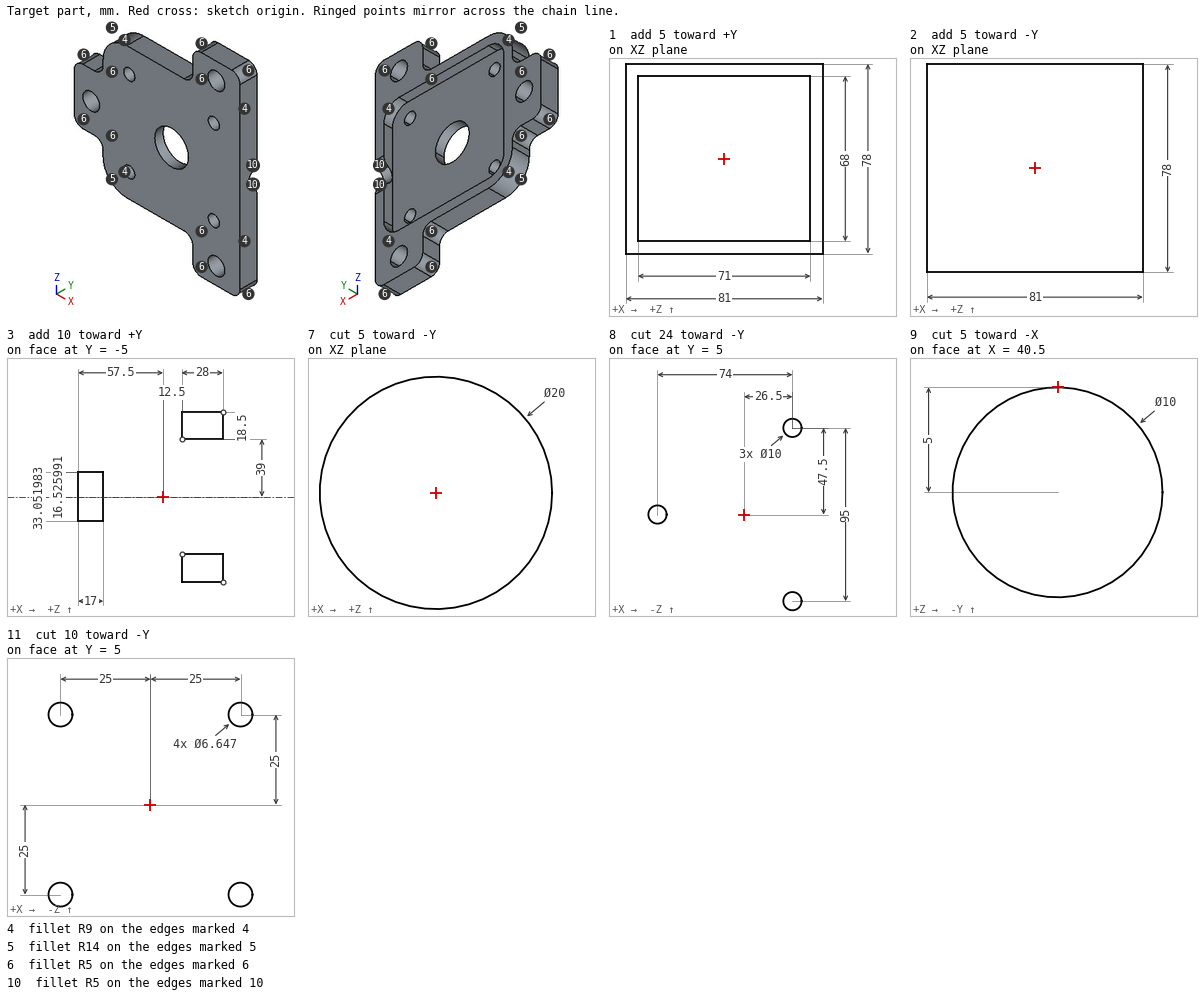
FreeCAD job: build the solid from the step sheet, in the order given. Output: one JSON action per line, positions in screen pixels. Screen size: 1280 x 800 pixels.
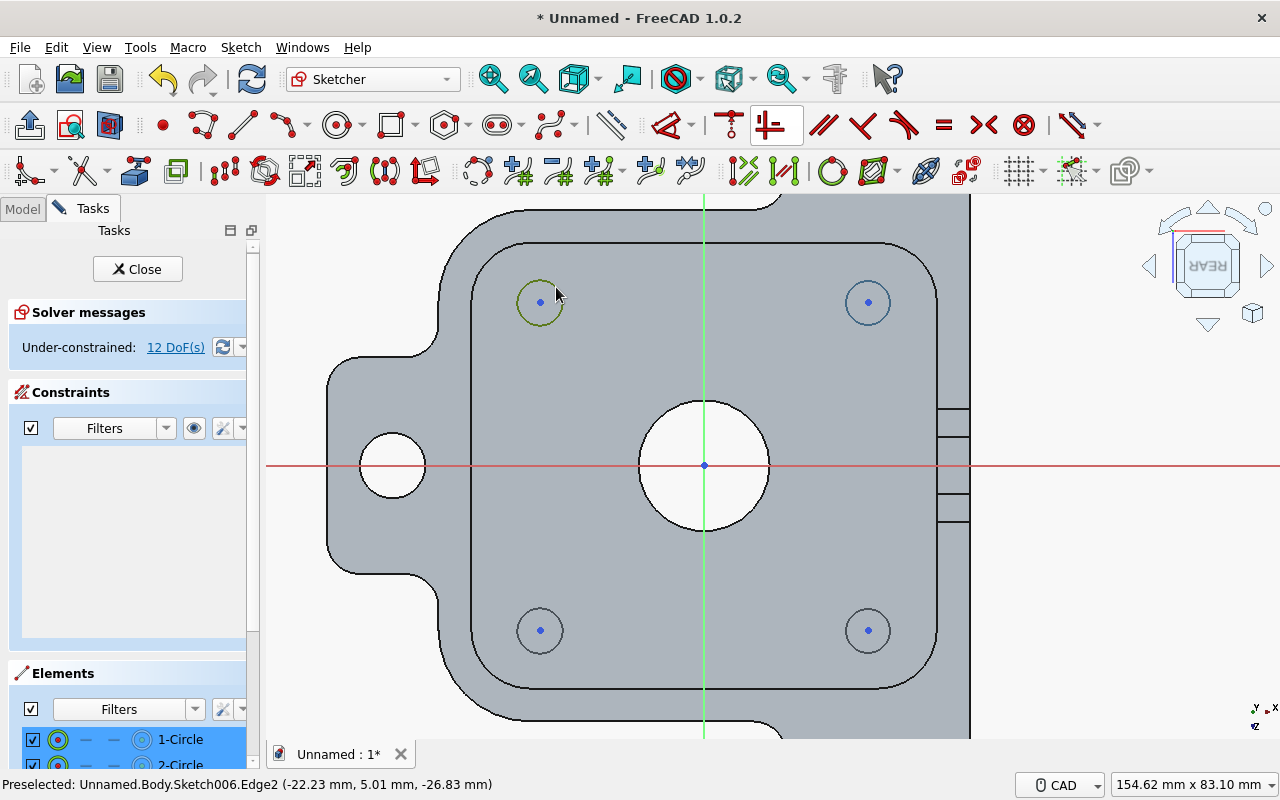
{"action": "left_click", "coordinate": [556, 615]}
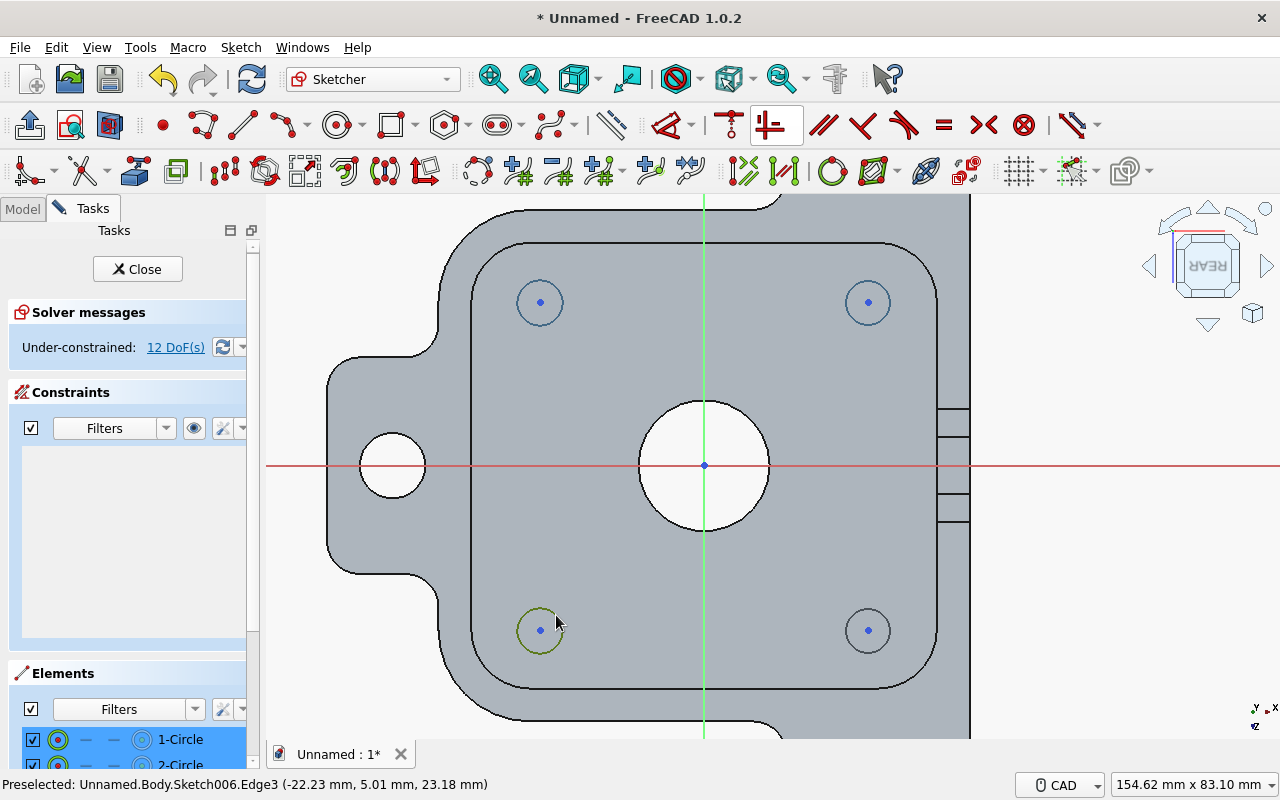
{"action": "left_click", "coordinate": [883, 615]}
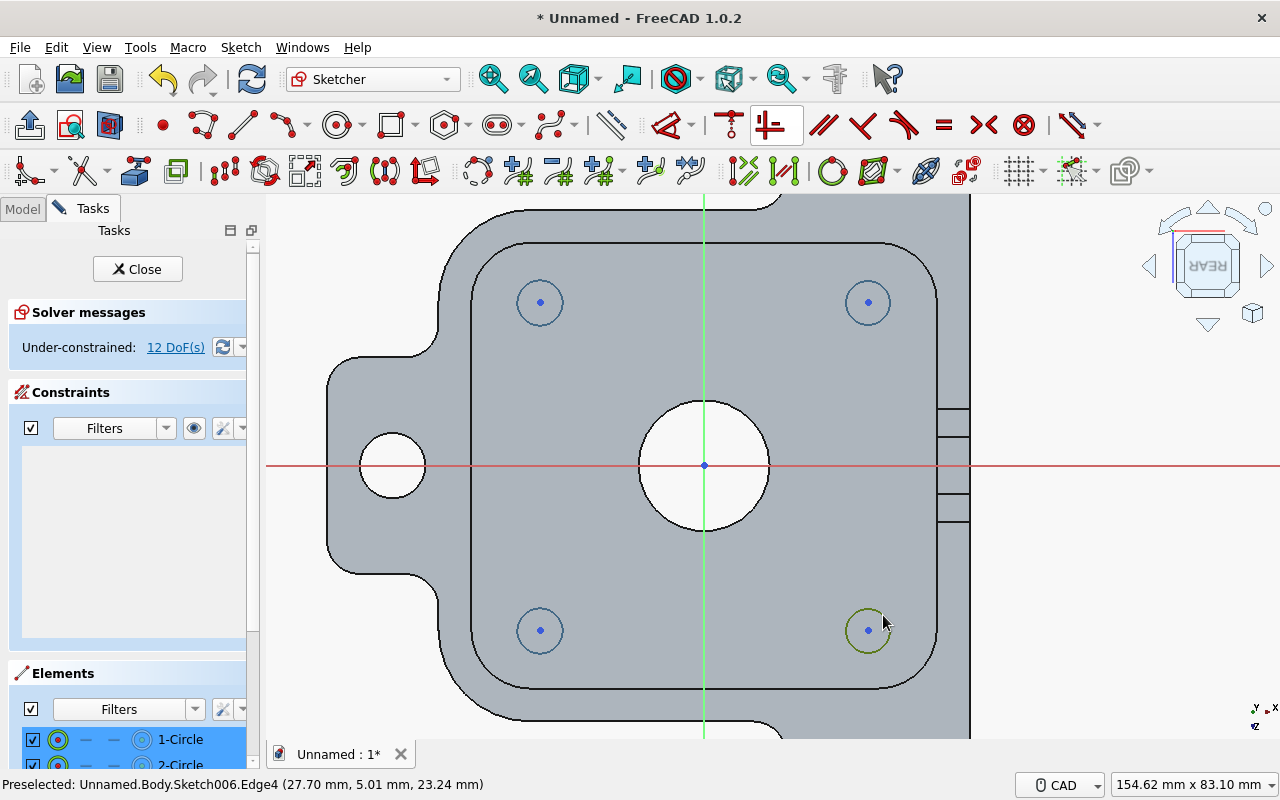
{"action": "key", "text": "e"}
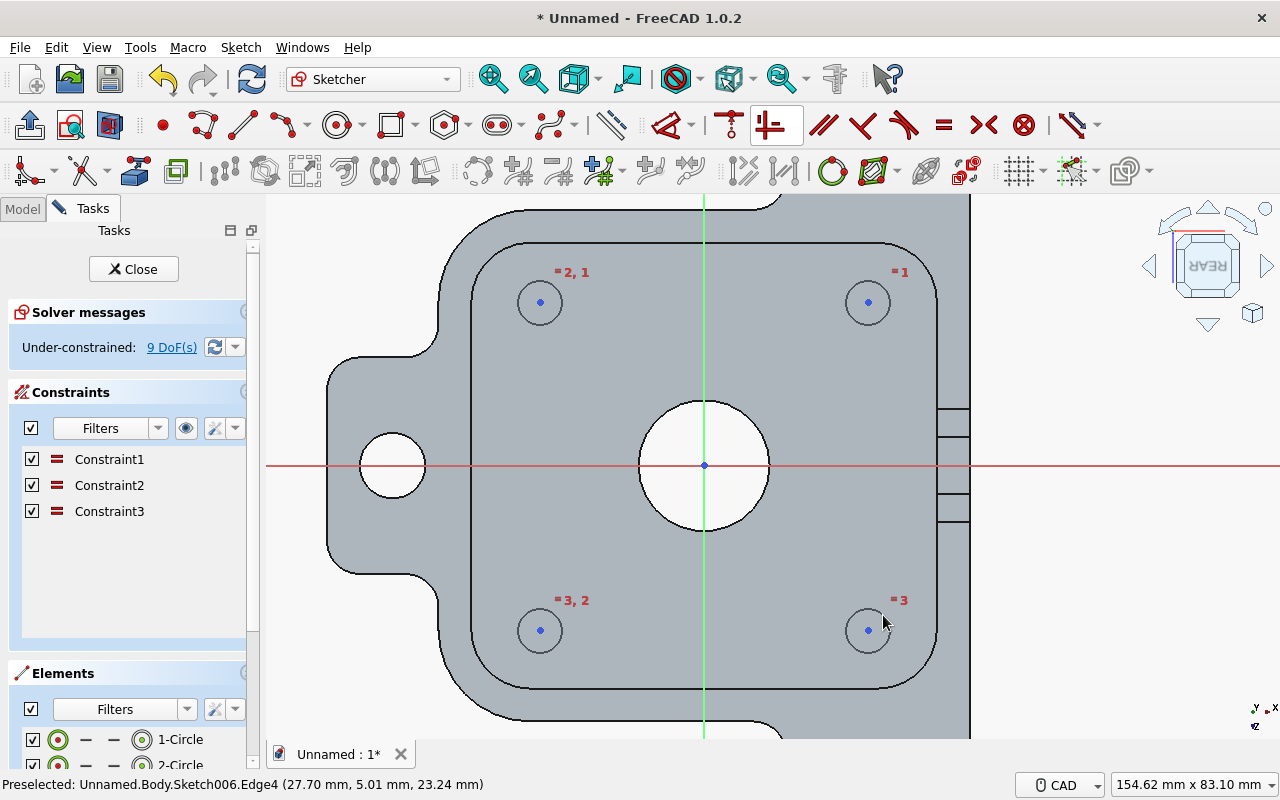
{"action": "left_click", "coordinate": [868, 303]}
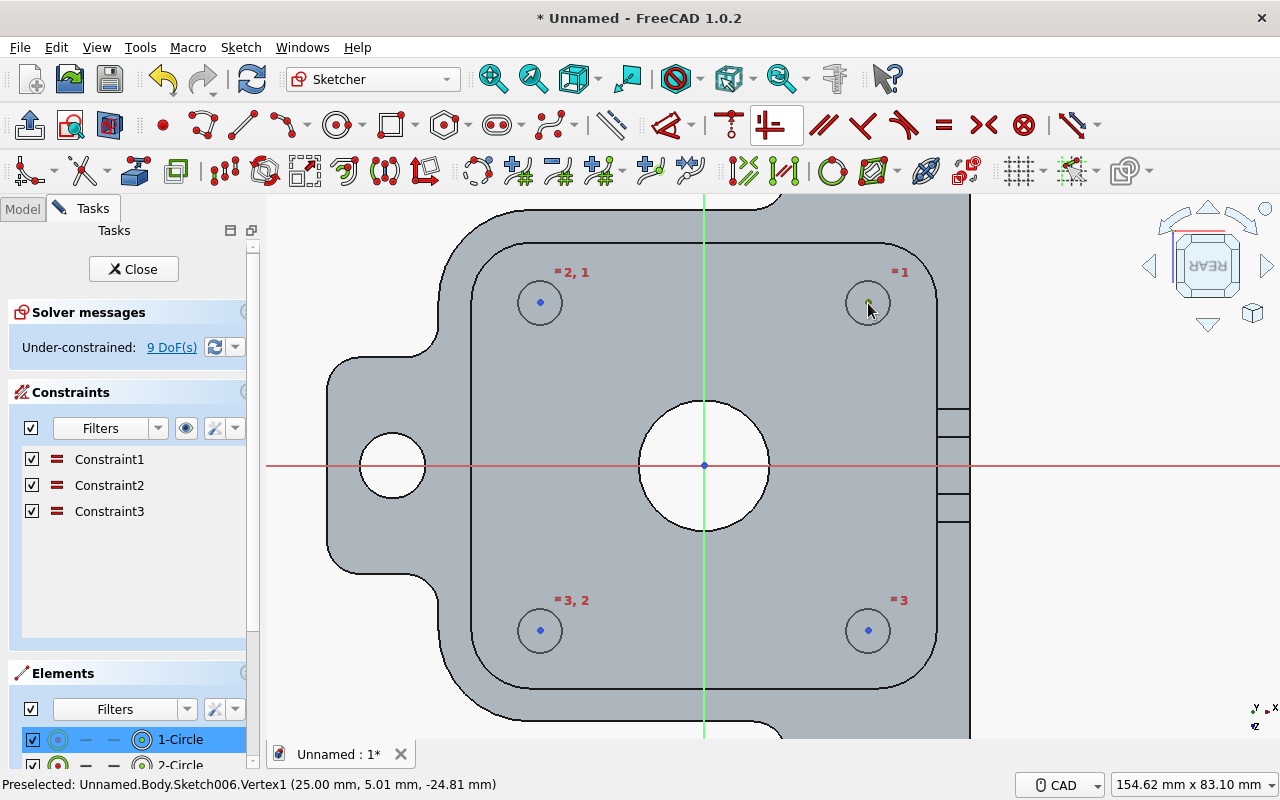
{"action": "left_click", "coordinate": [540, 303]}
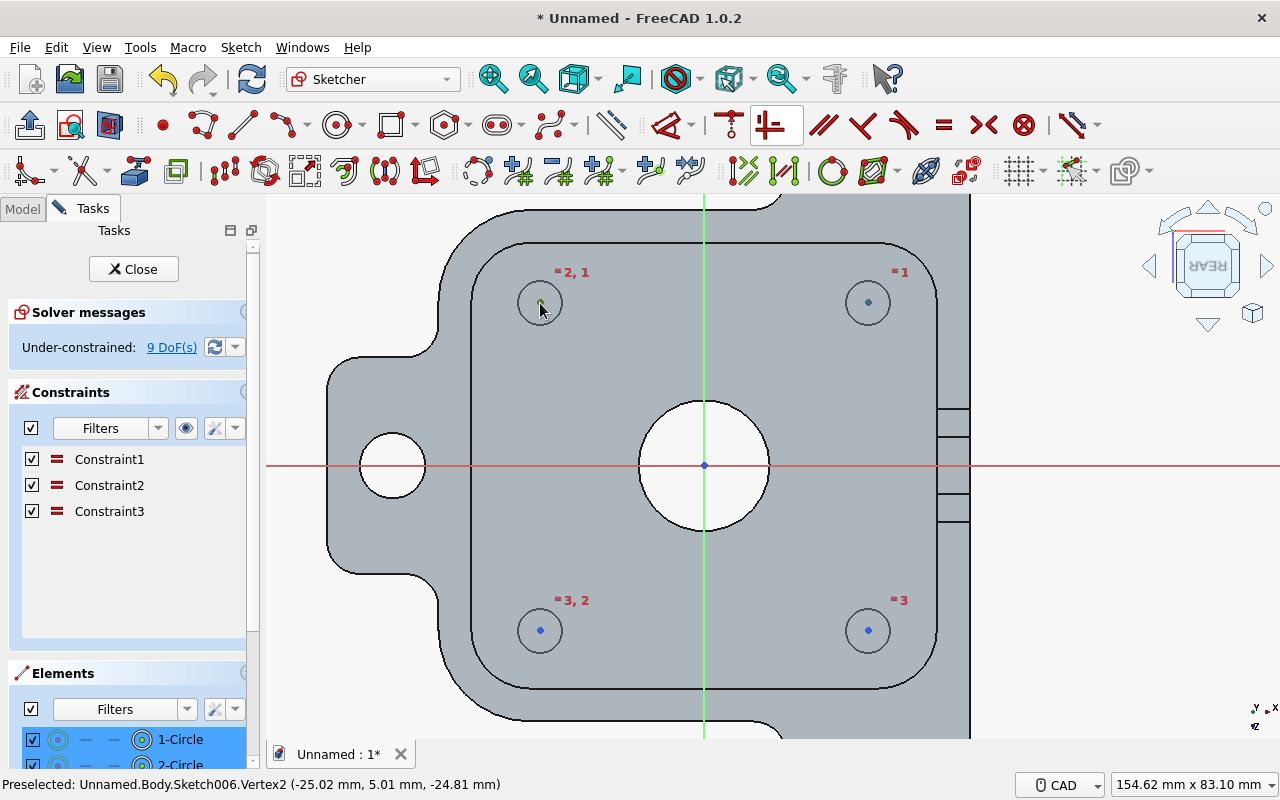
{"action": "key", "text": "h"}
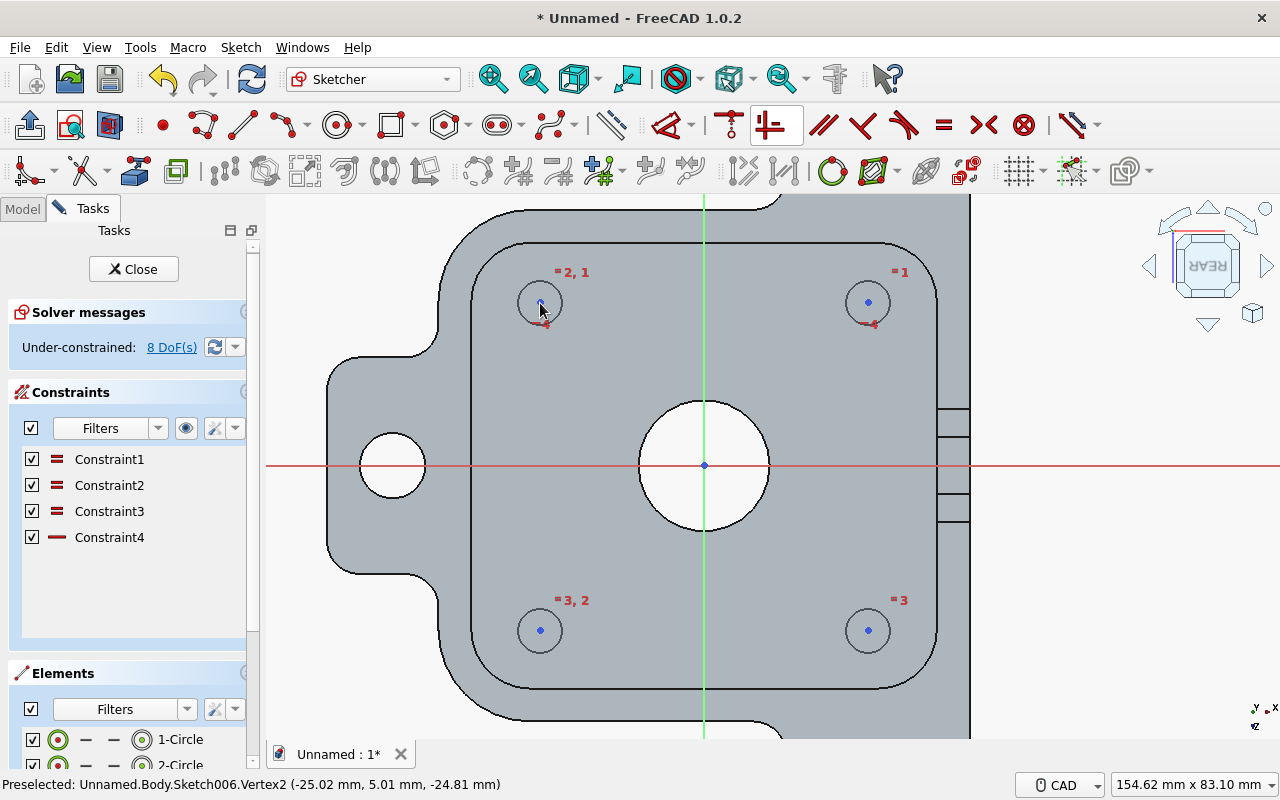
{"action": "left_click", "coordinate": [540, 303]}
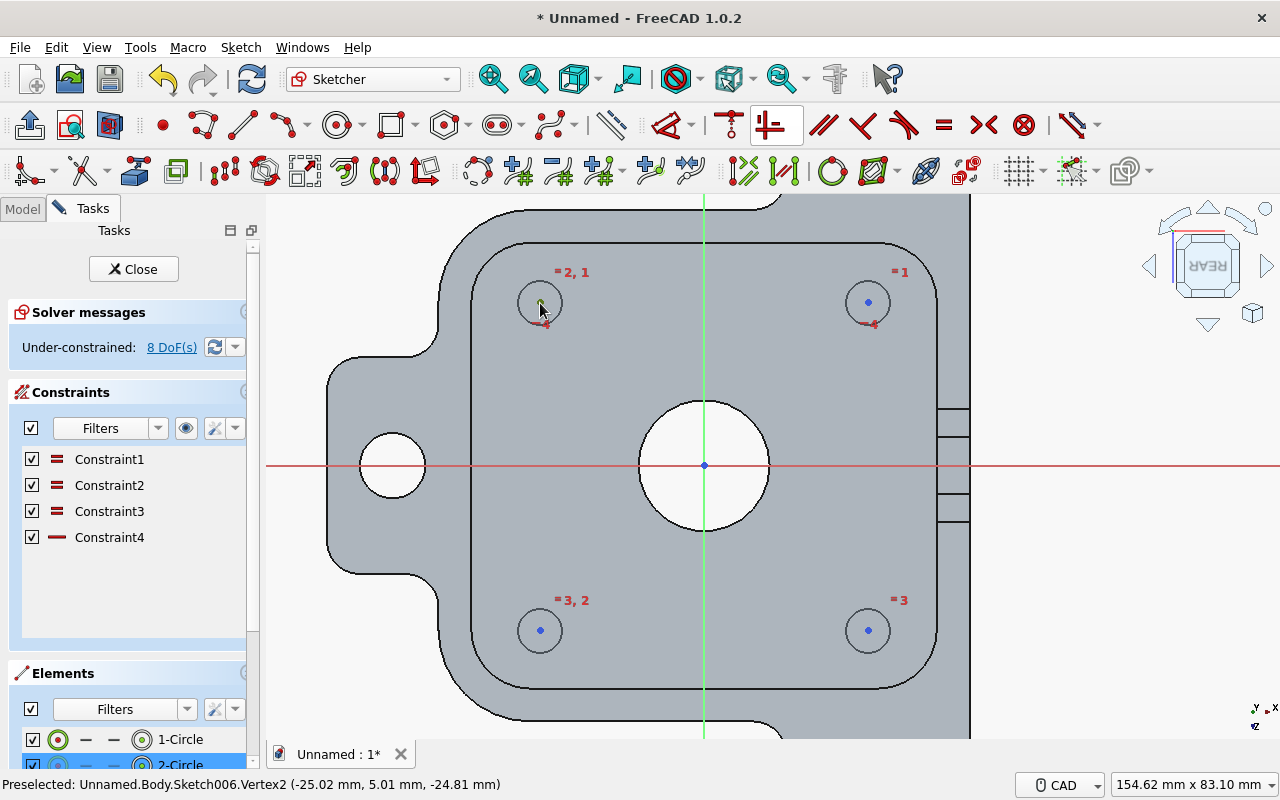
{"action": "left_click", "coordinate": [540, 631]}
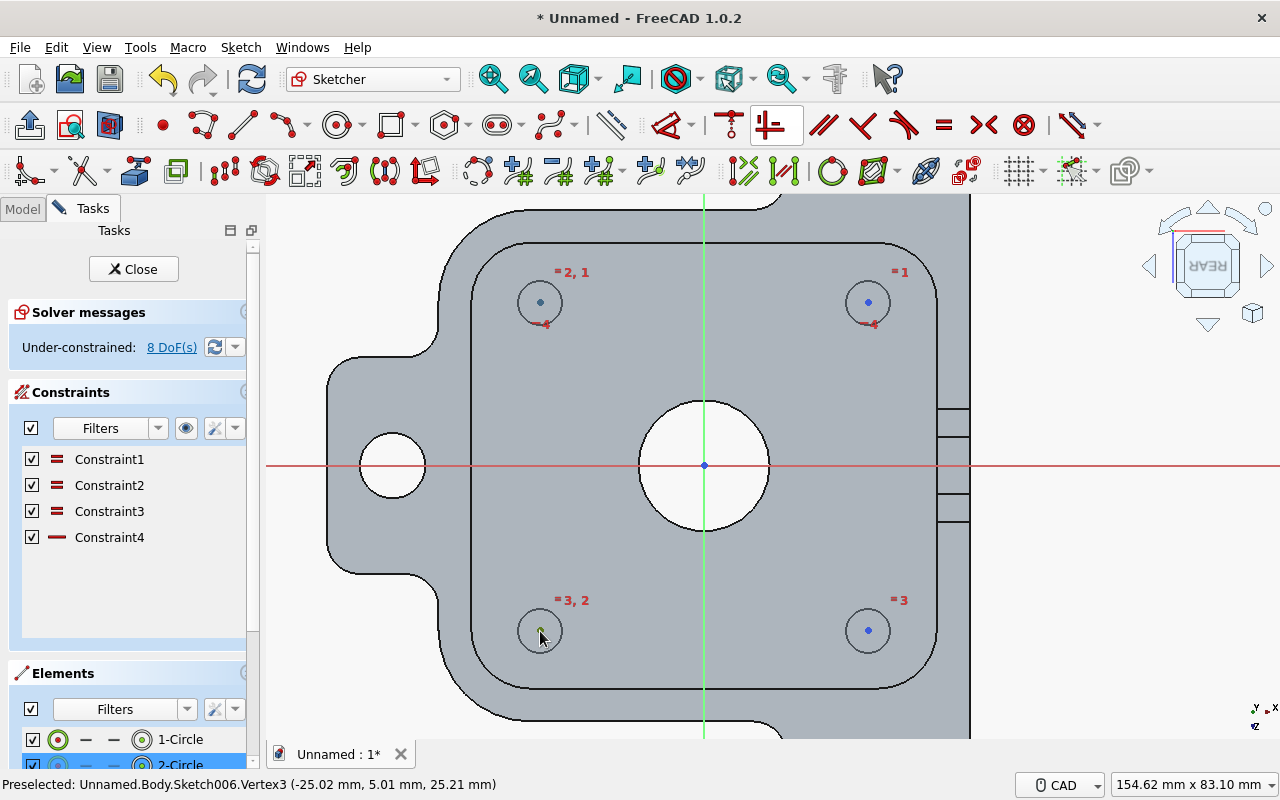
{"action": "key", "text": "v"}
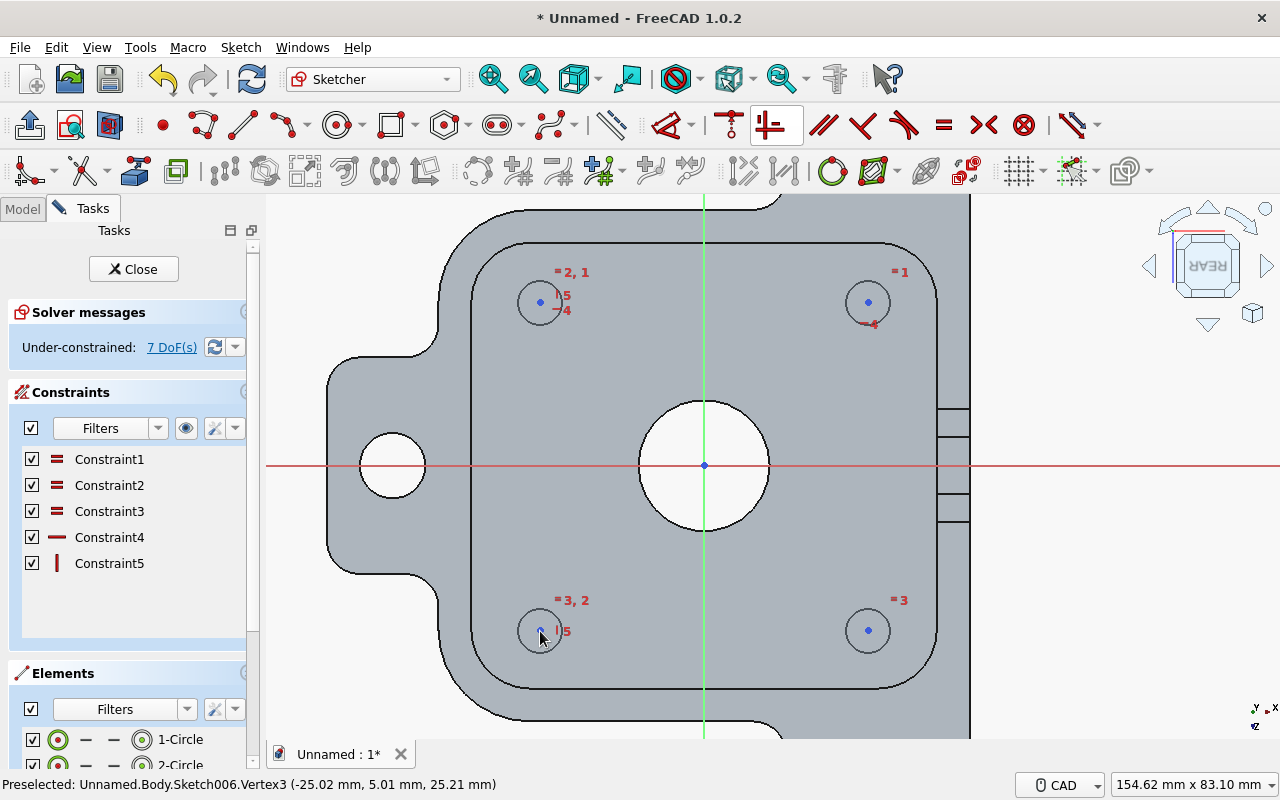
{"action": "left_click", "coordinate": [868, 303]}